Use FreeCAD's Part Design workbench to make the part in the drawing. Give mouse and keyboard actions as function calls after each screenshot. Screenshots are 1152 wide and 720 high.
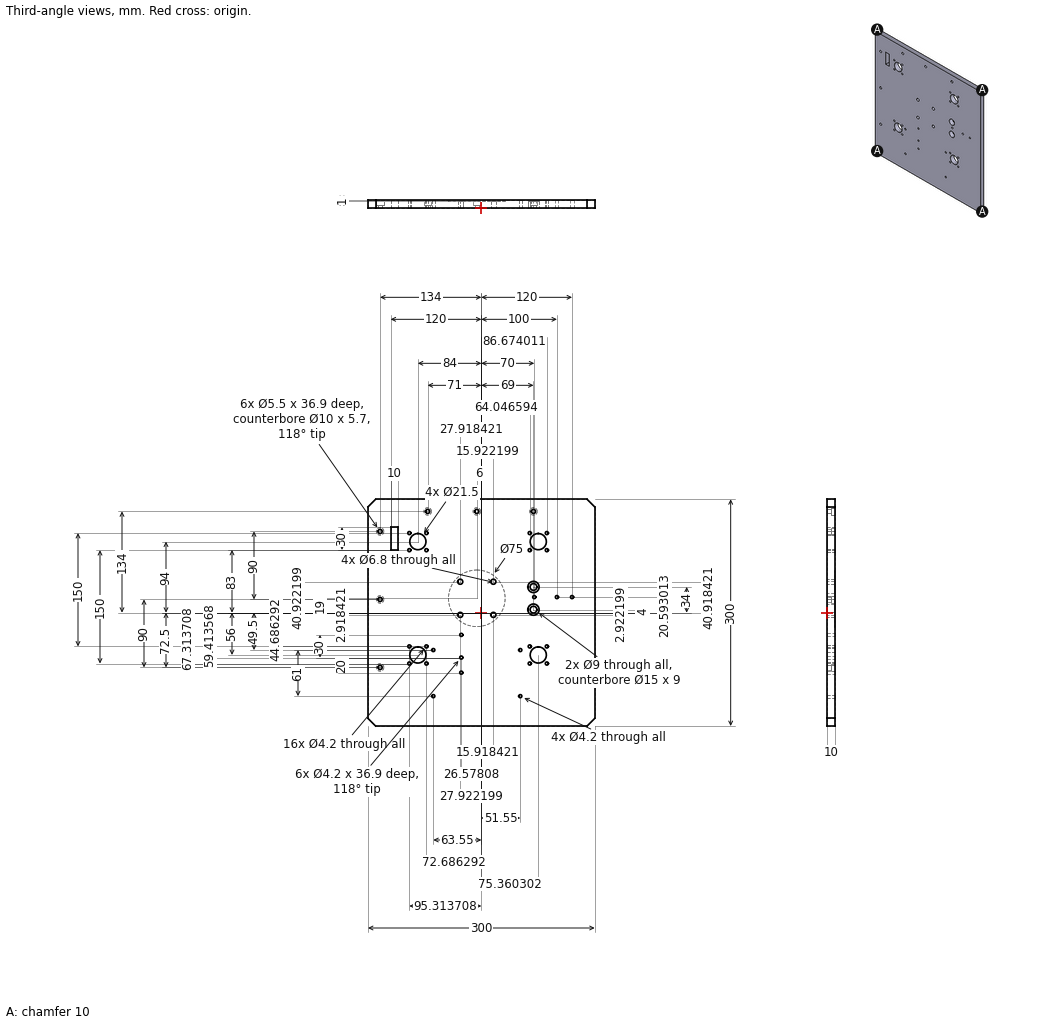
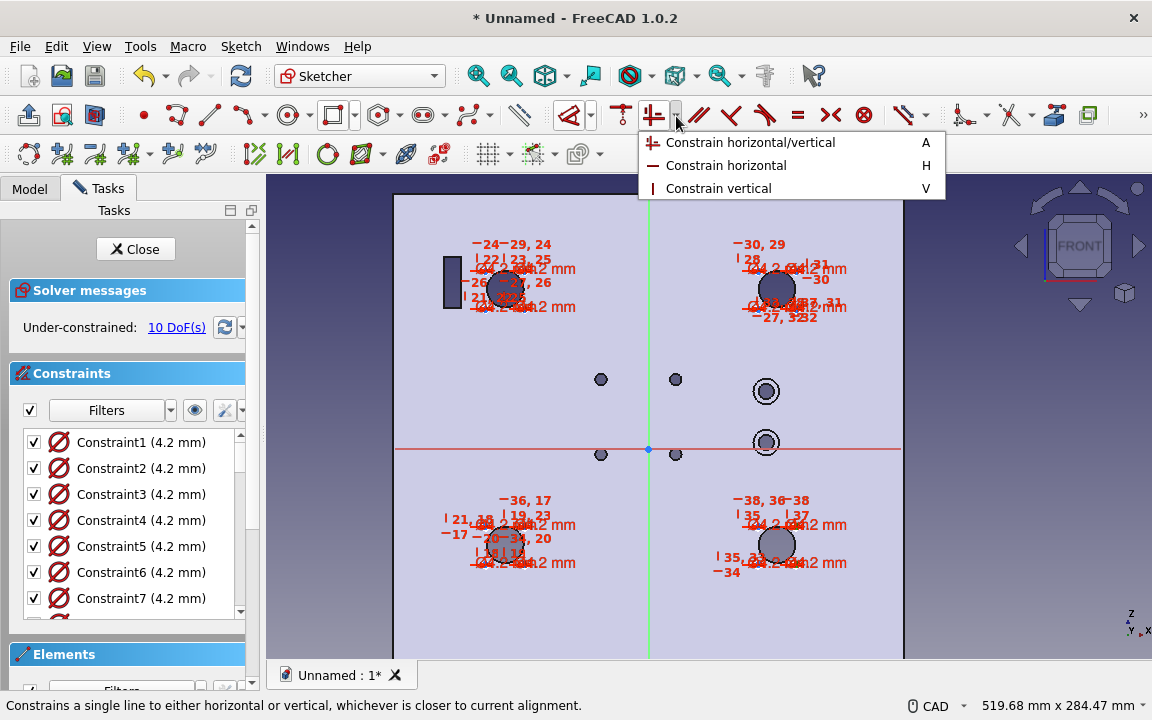
click(792, 188)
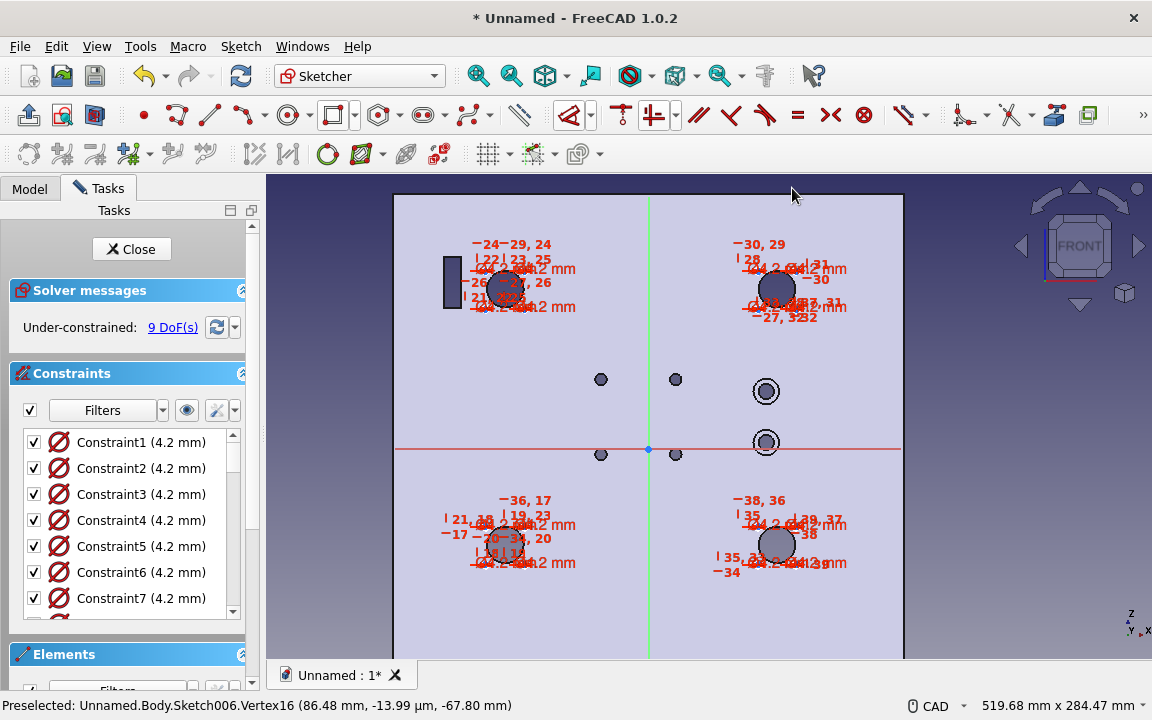
click(758, 565)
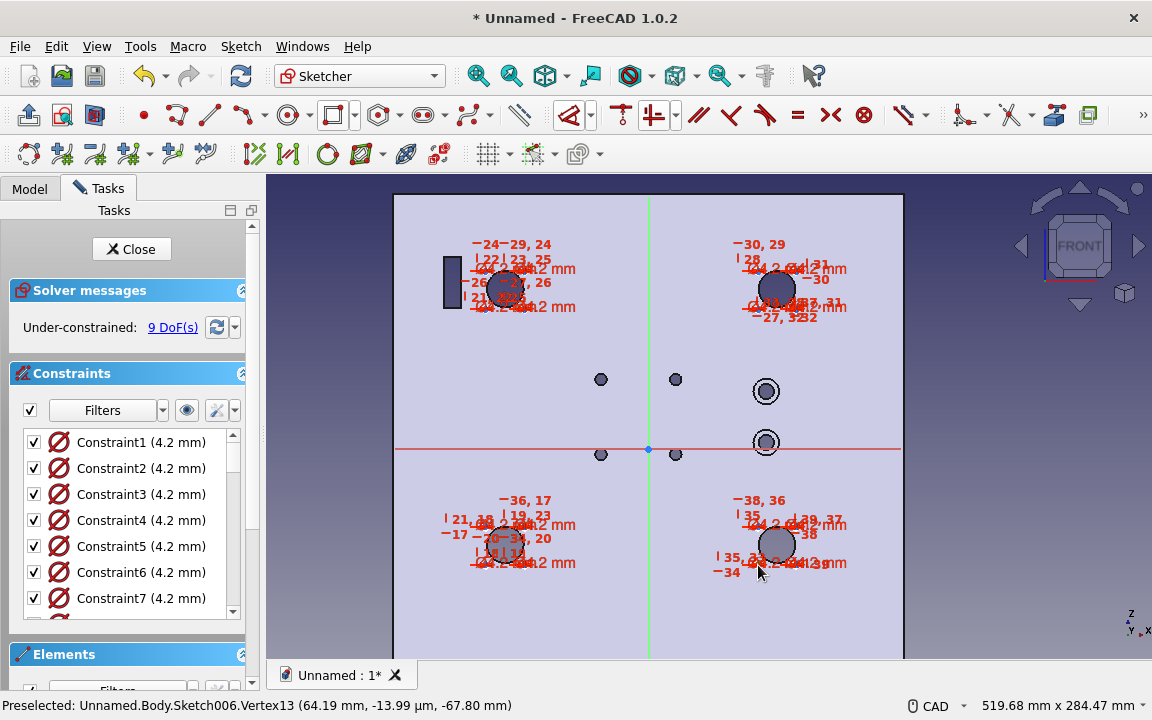
click(796, 565)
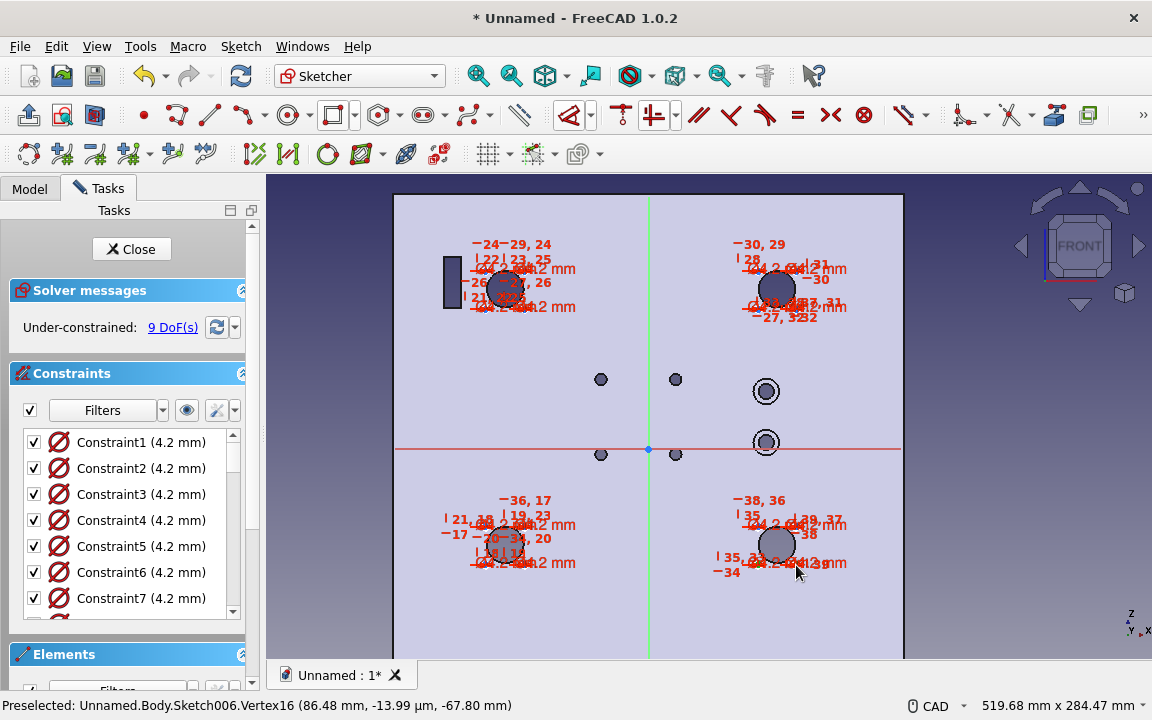
click(676, 116)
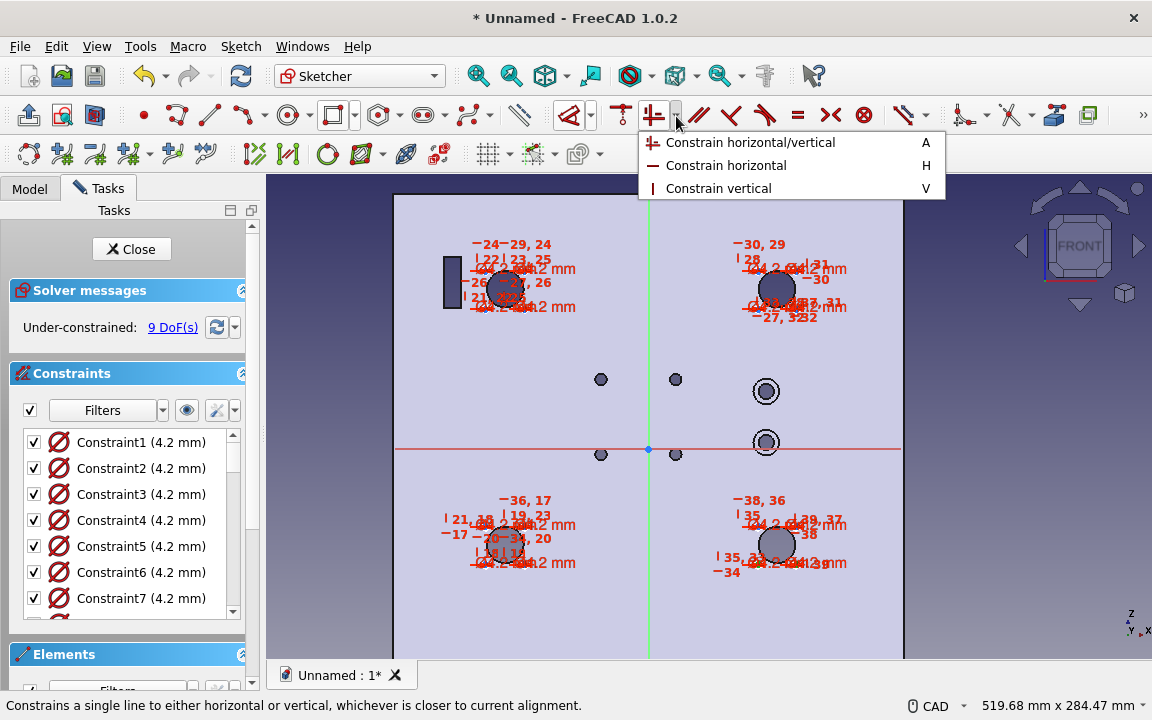
click(792, 166)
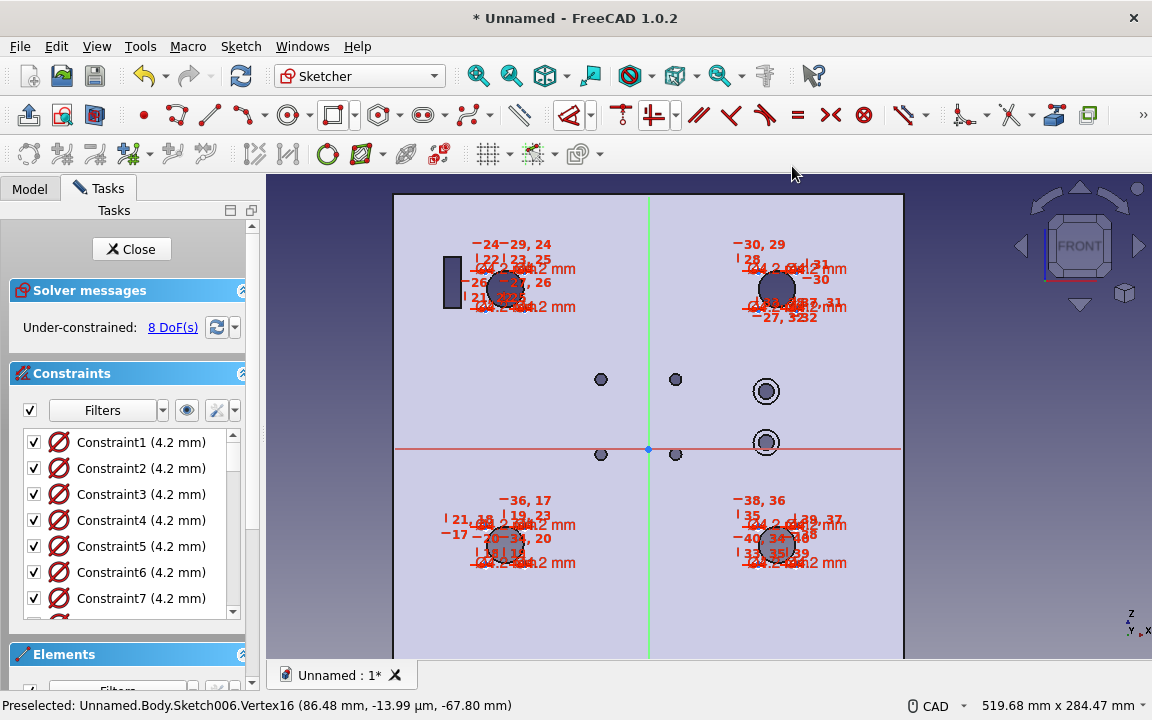
click(486, 565)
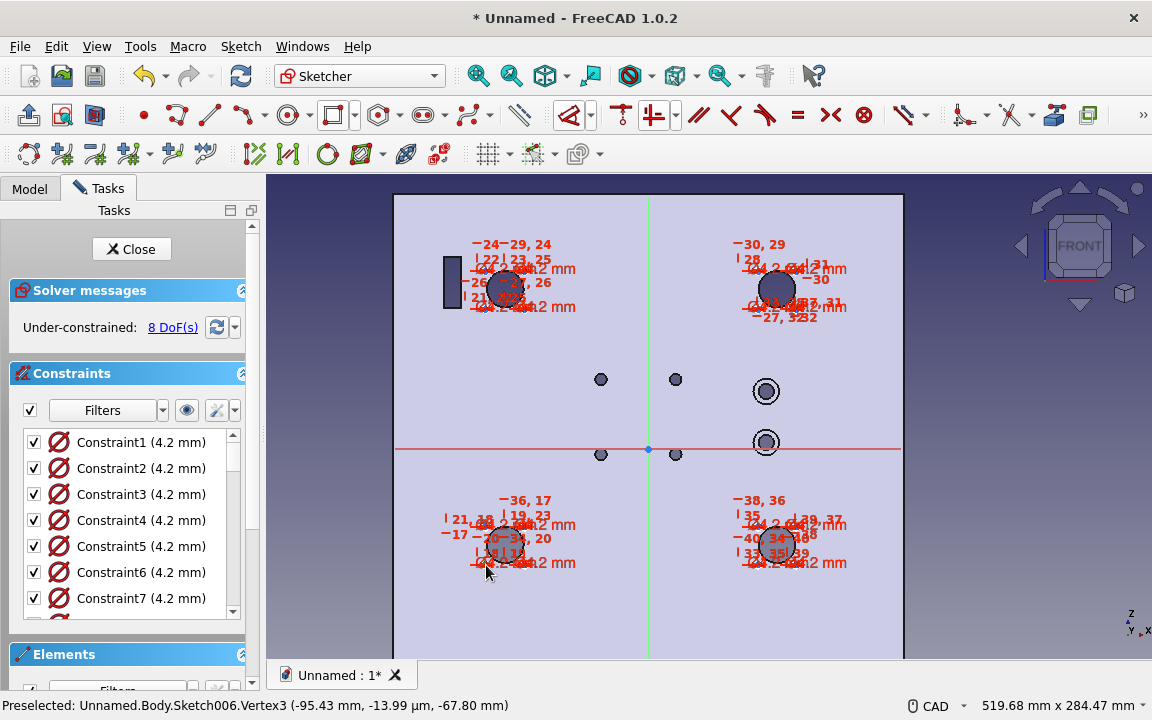
click(486, 309)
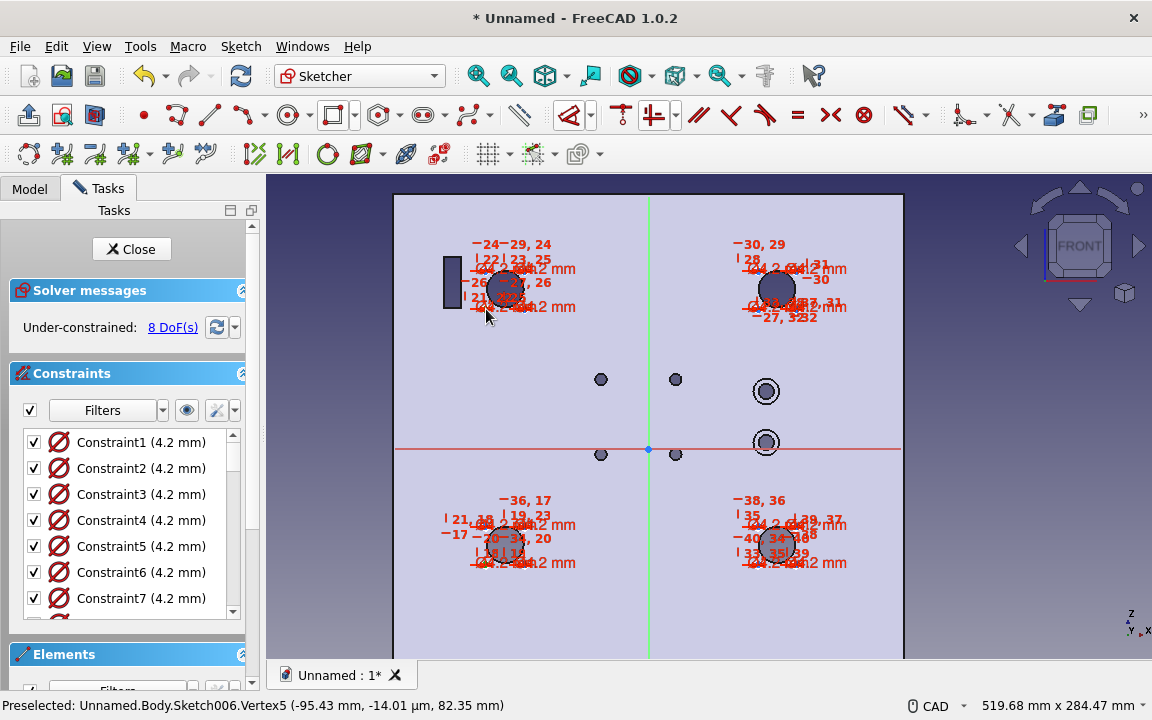
key(i)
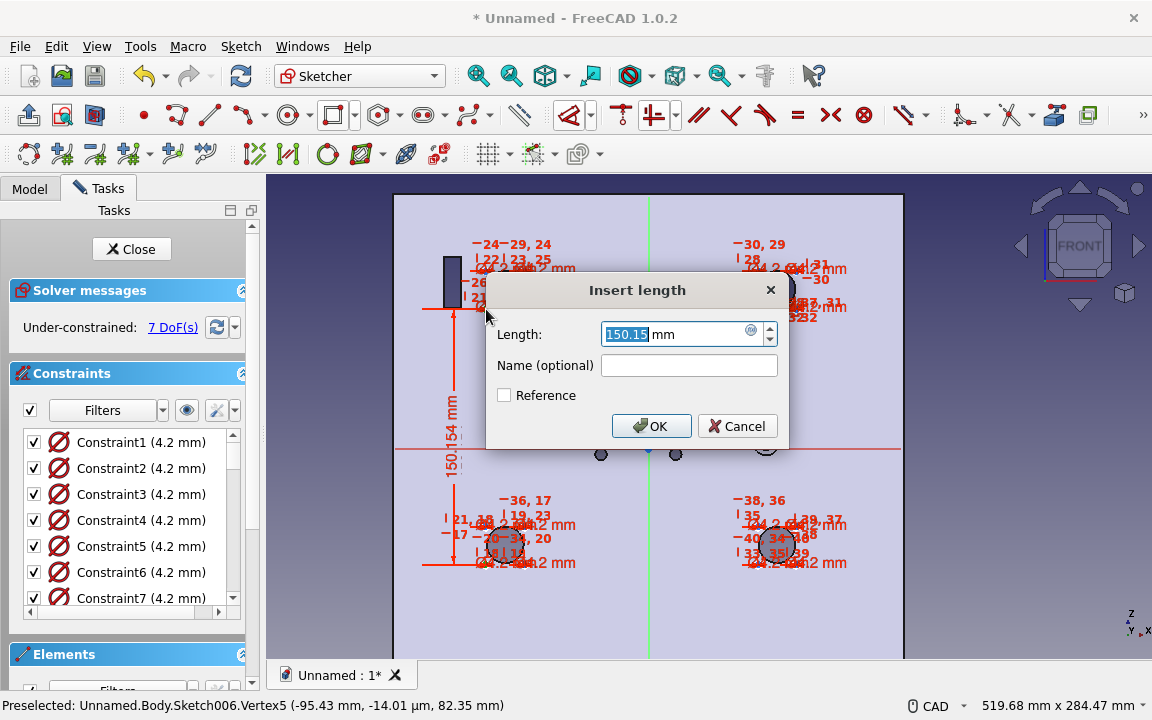
text(150)
key(Return)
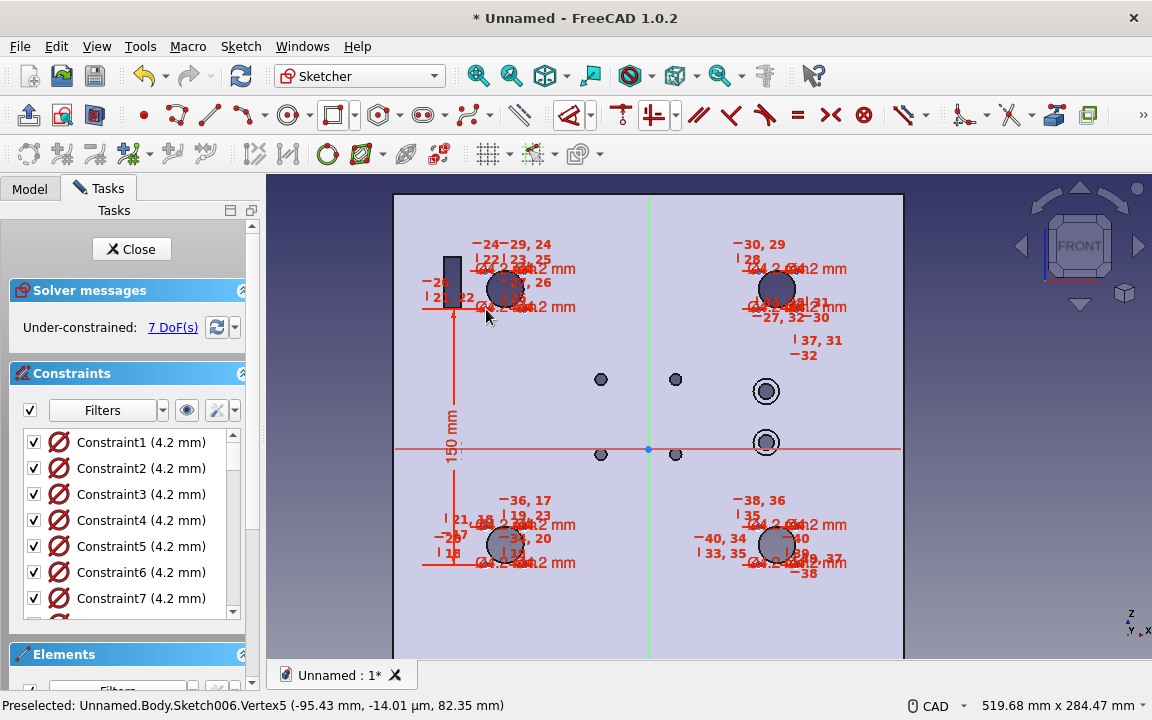
click(486, 527)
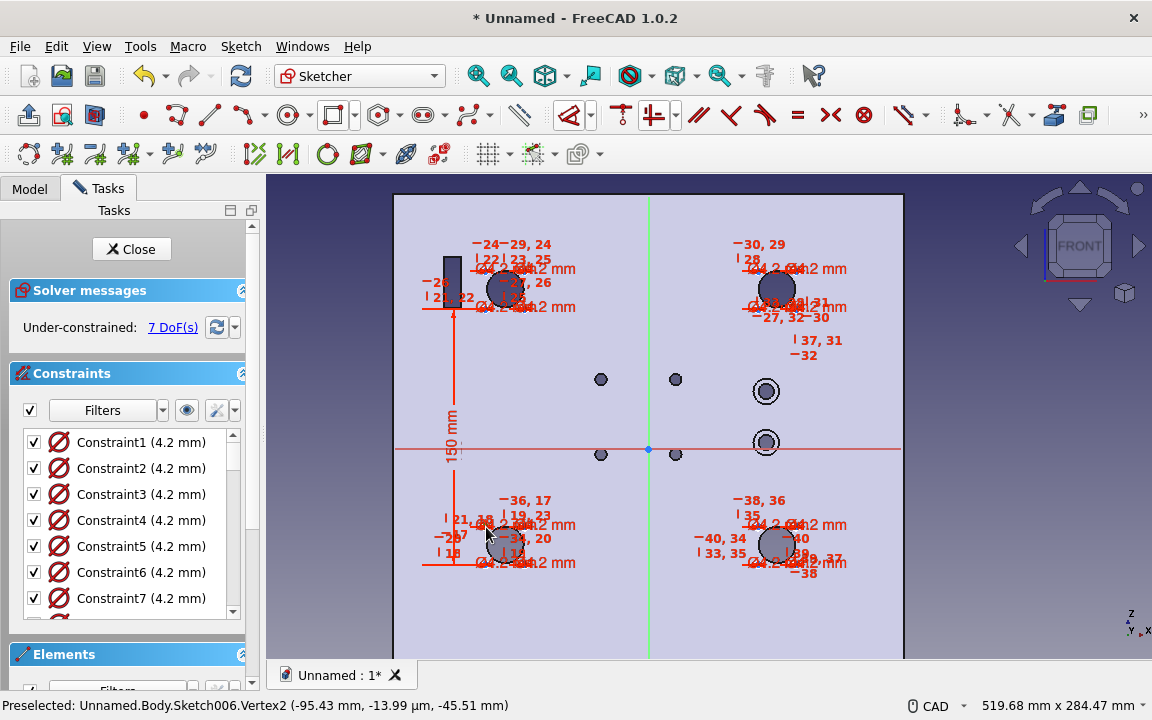
click(486, 271)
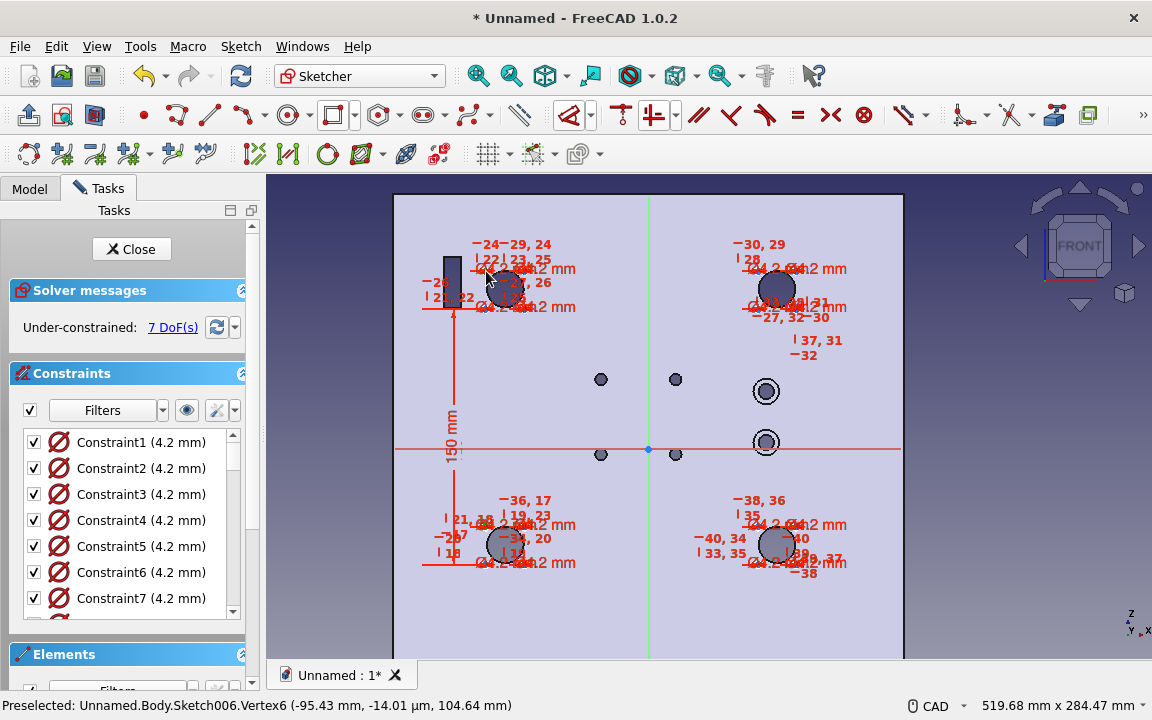
key(i)